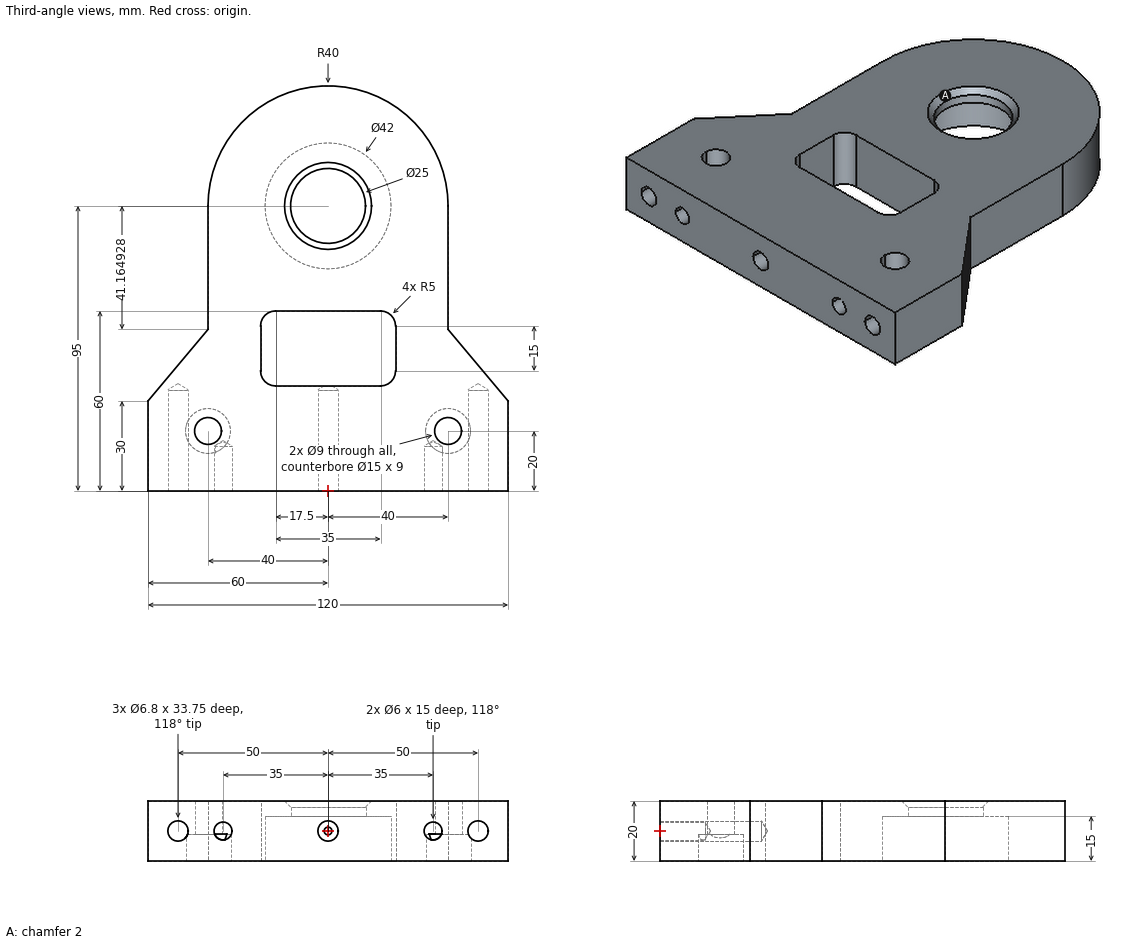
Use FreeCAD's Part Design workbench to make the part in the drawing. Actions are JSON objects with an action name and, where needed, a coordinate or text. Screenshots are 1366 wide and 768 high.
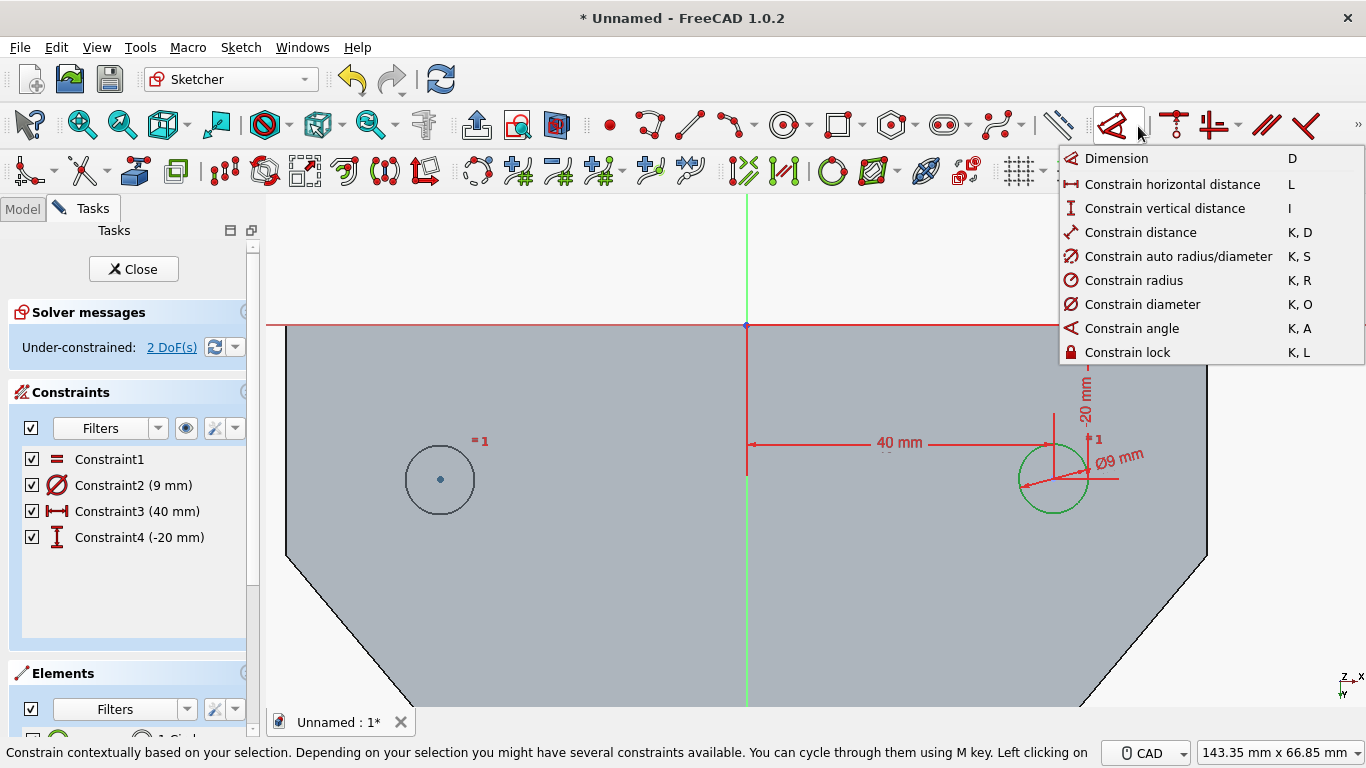
{"action": "left_click", "coordinate": [1212, 184]}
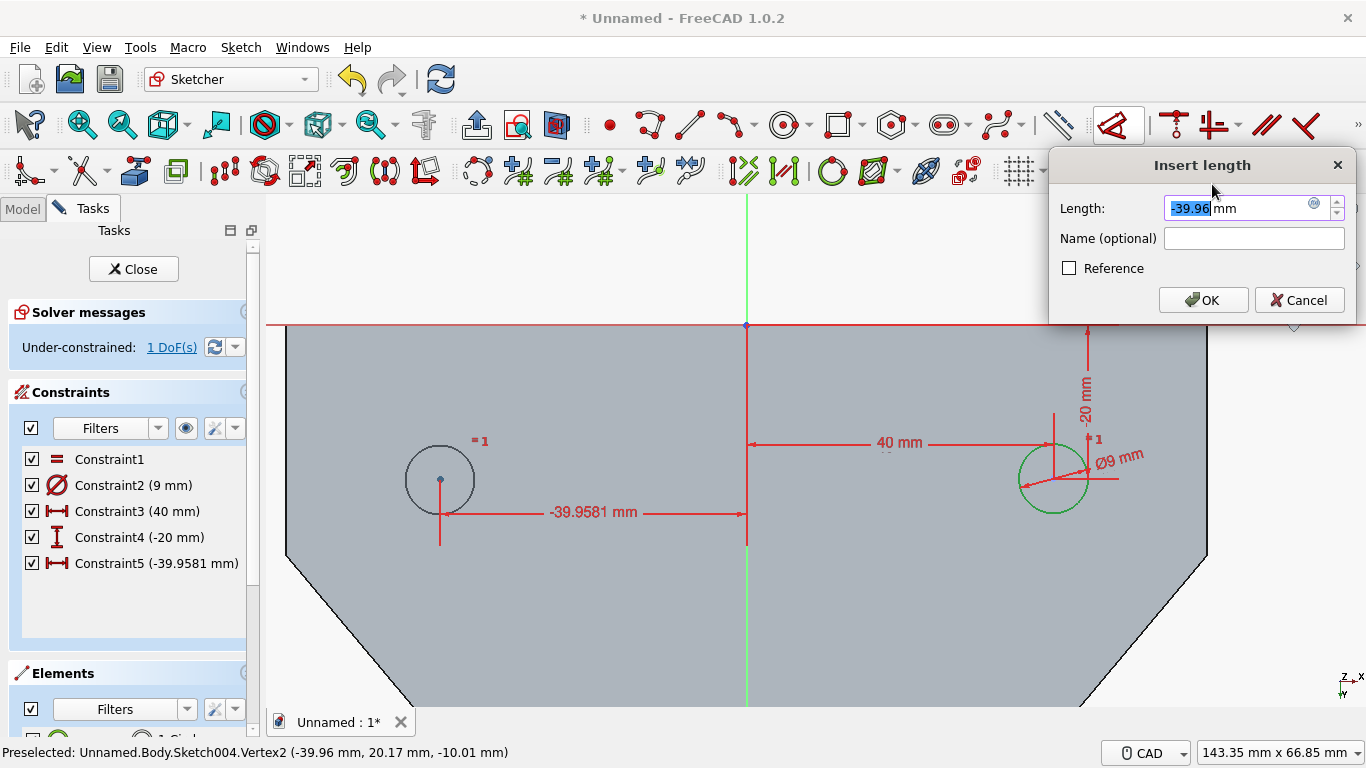
{"action": "type", "text": "-40"}
{"action": "key", "text": "Return"}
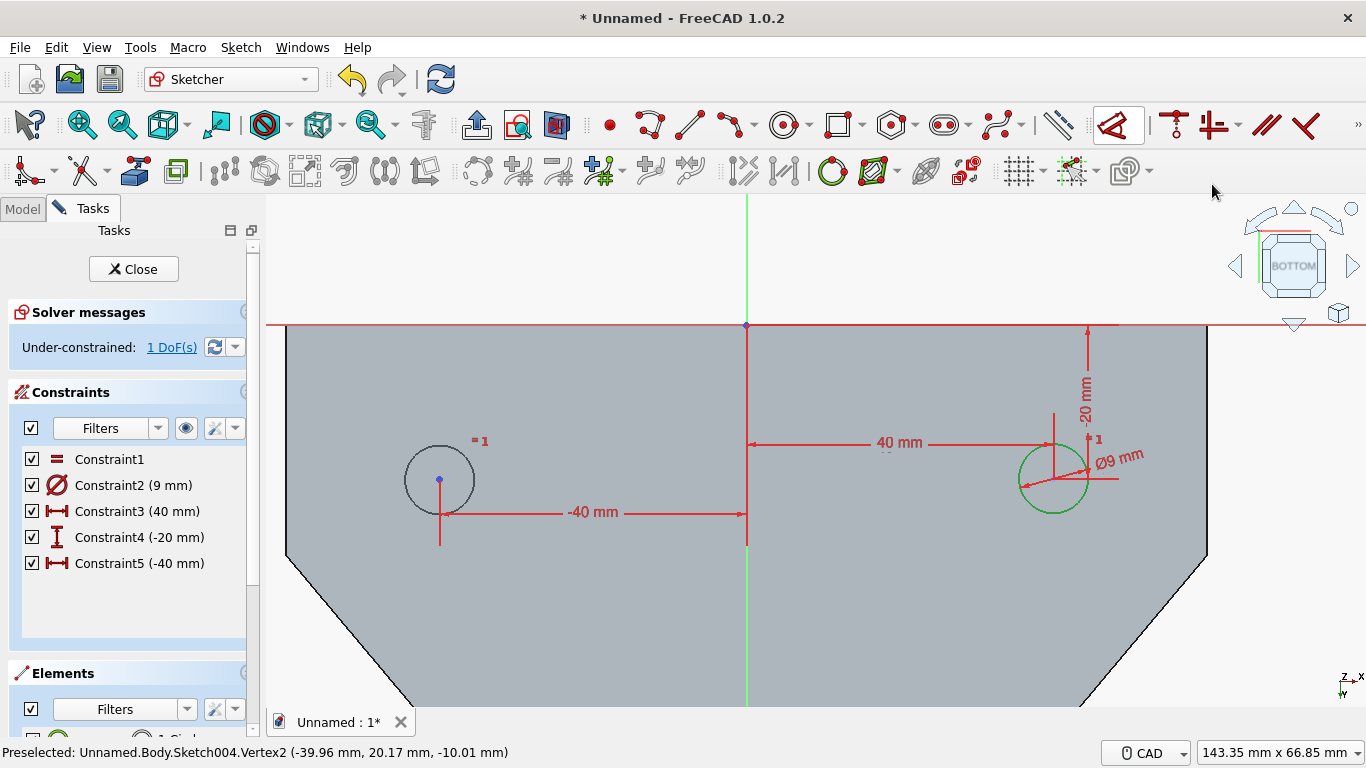
{"action": "left_click", "coordinate": [440, 480]}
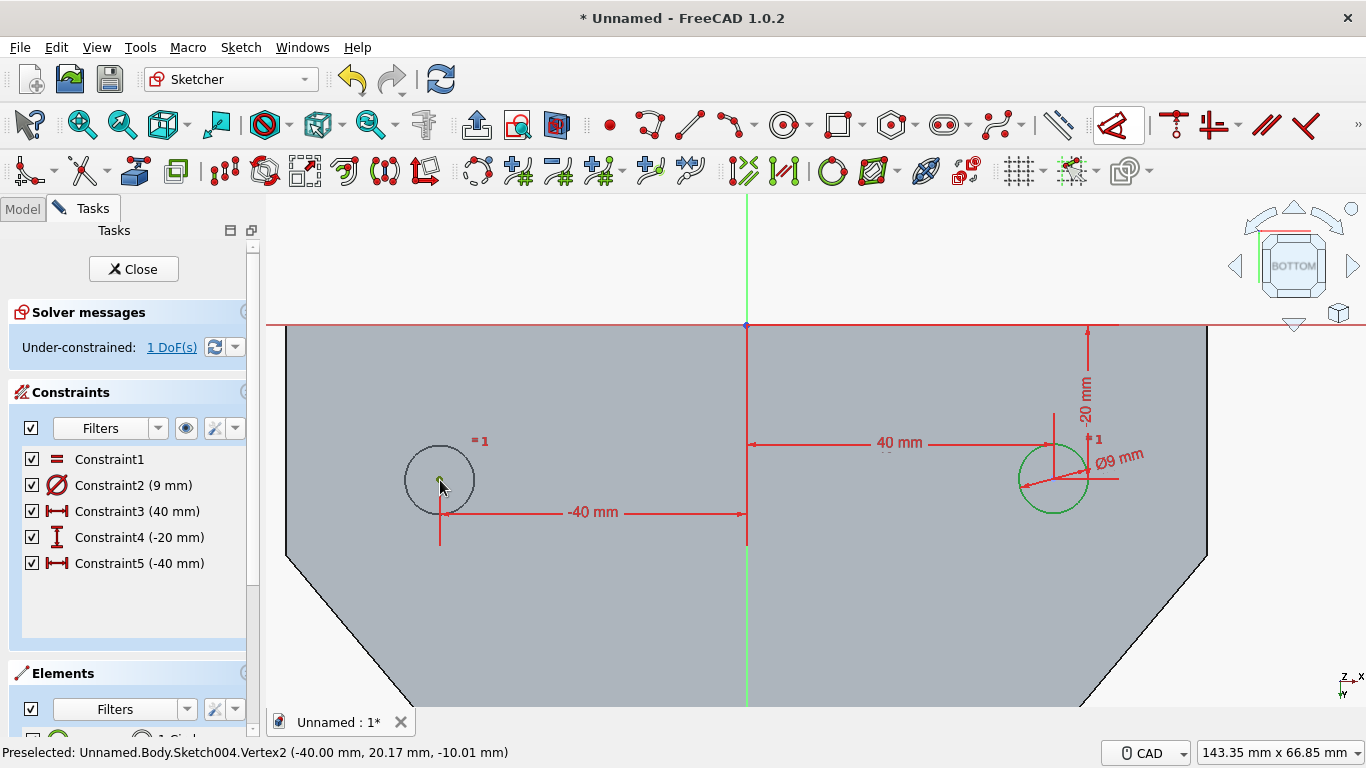
{"action": "key", "text": "i"}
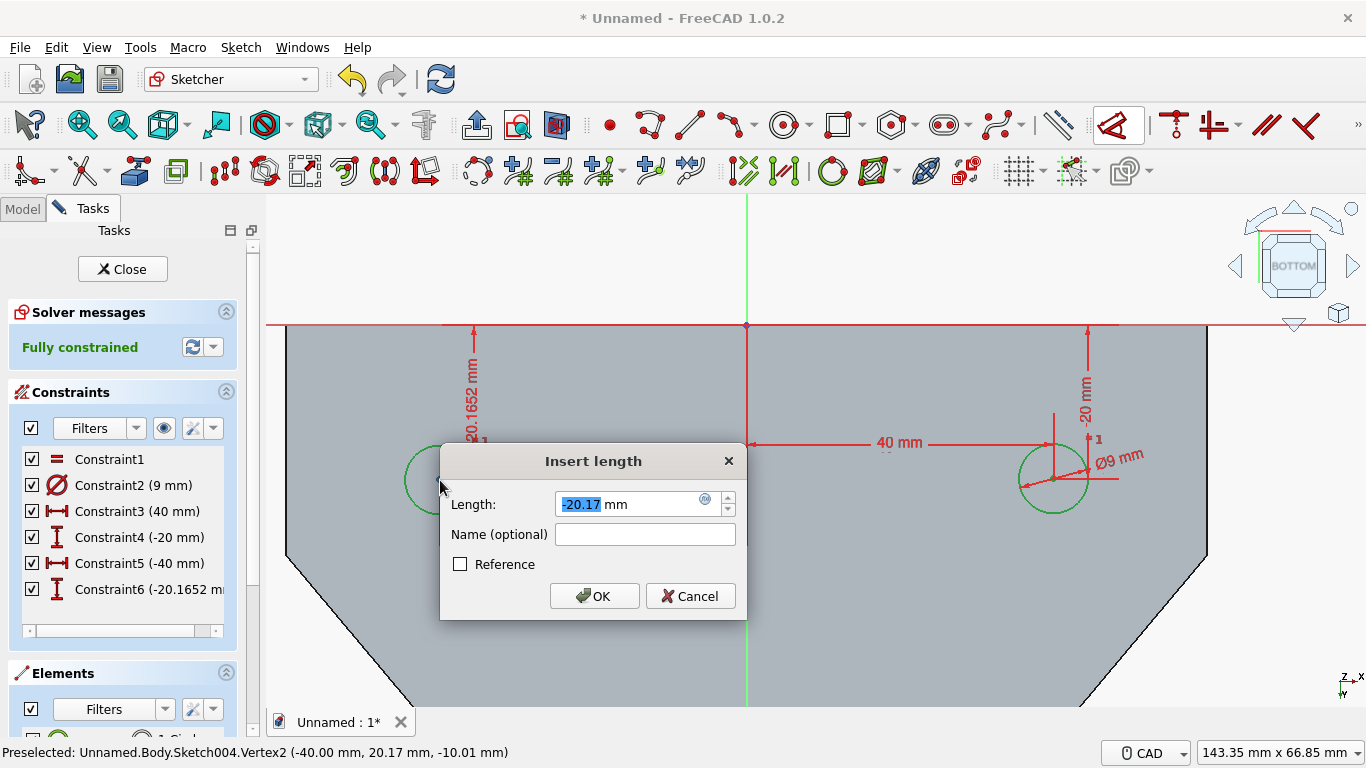
{"action": "type", "text": "-20"}
{"action": "key", "text": "Return"}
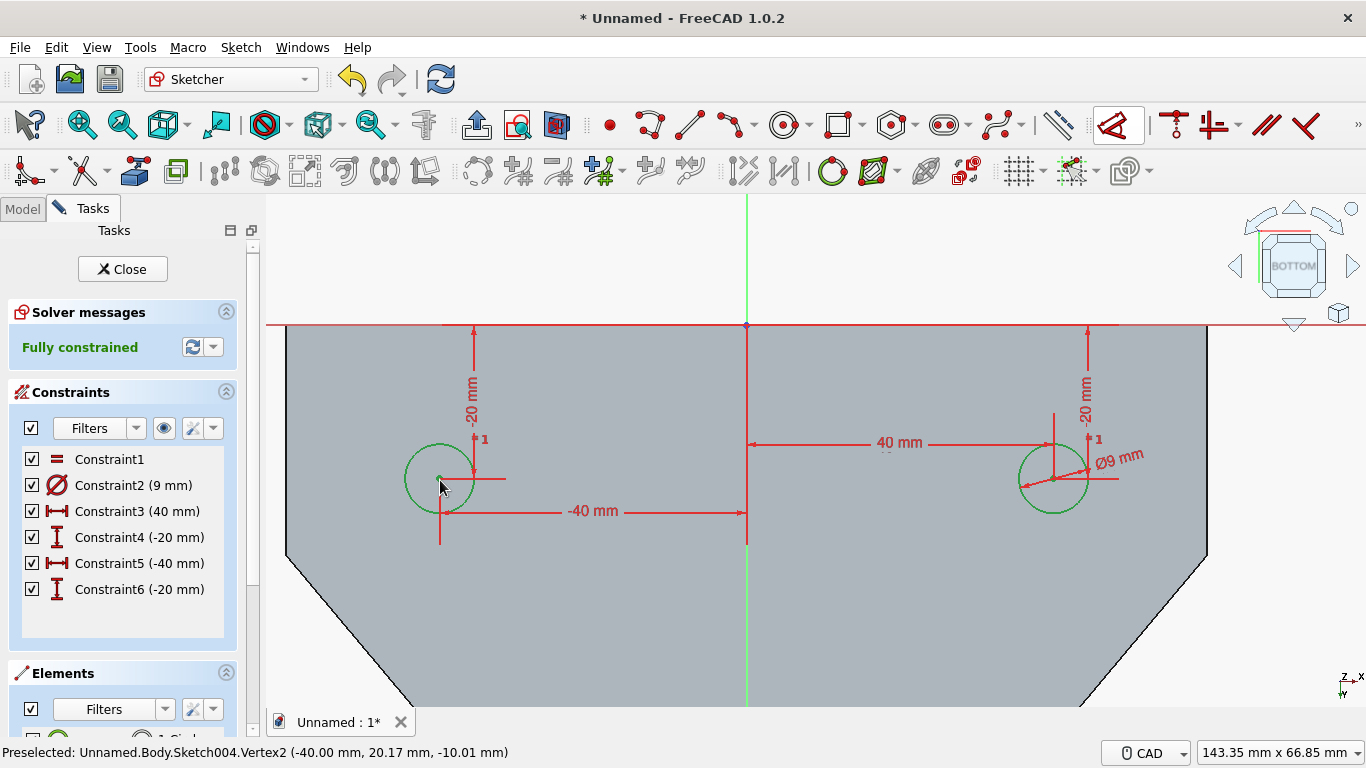
{"action": "left_click", "coordinate": [123, 269]}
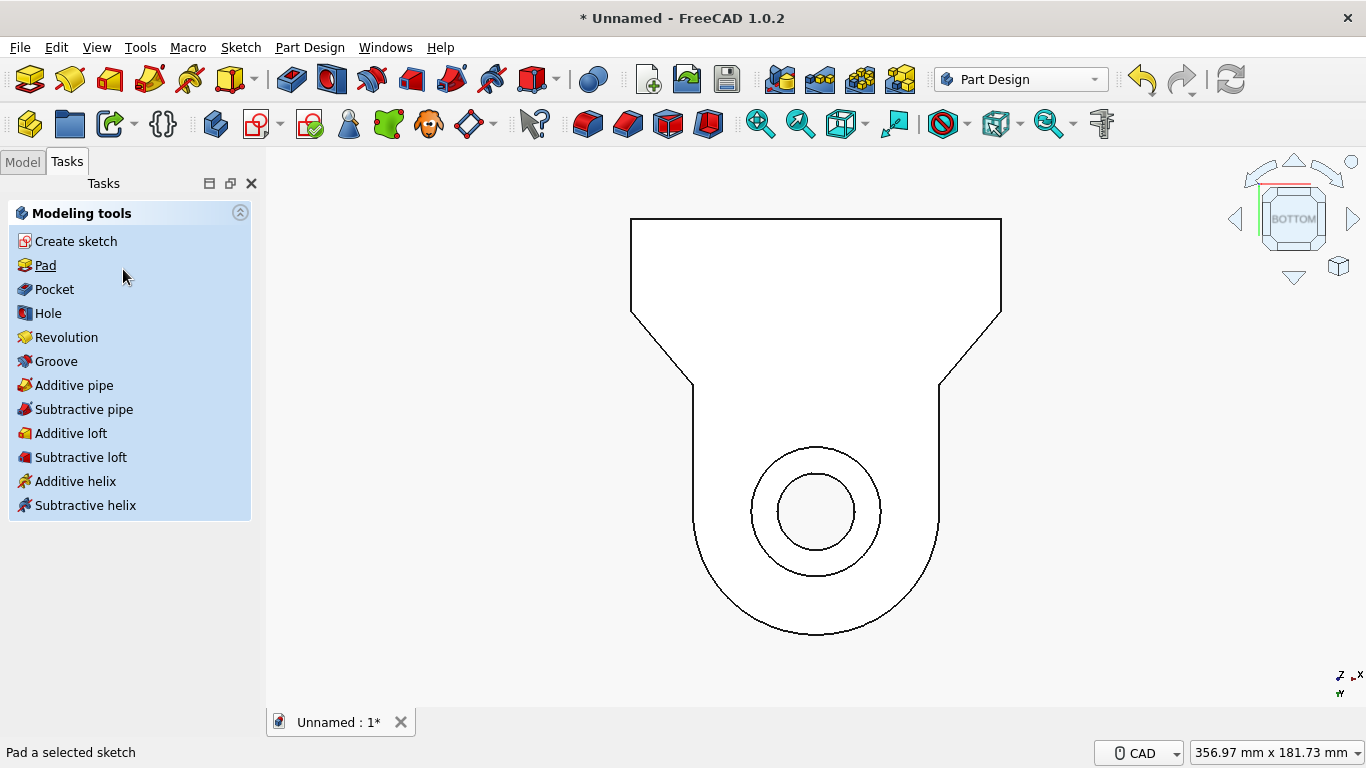
{"action": "left_click", "coordinate": [332, 80]}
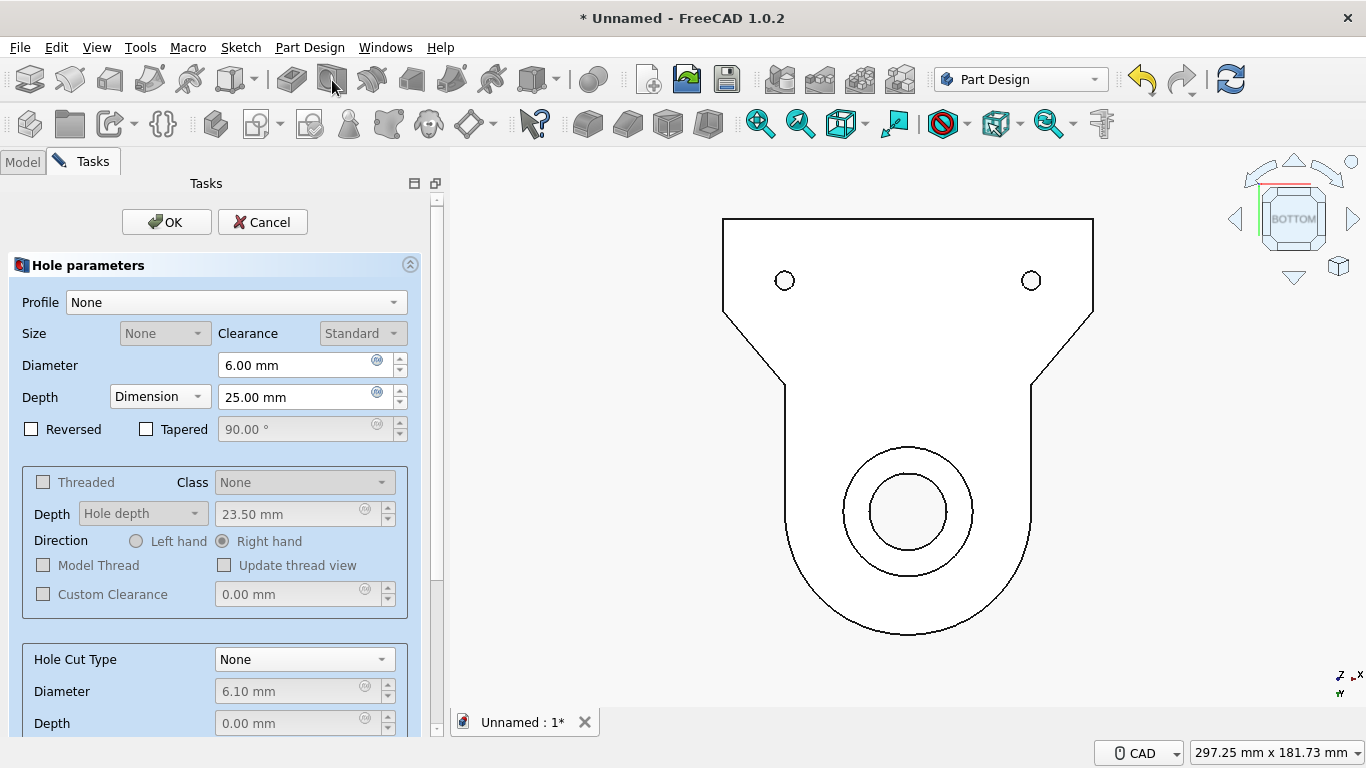
{"action": "triple_click", "coordinate": [305, 365]}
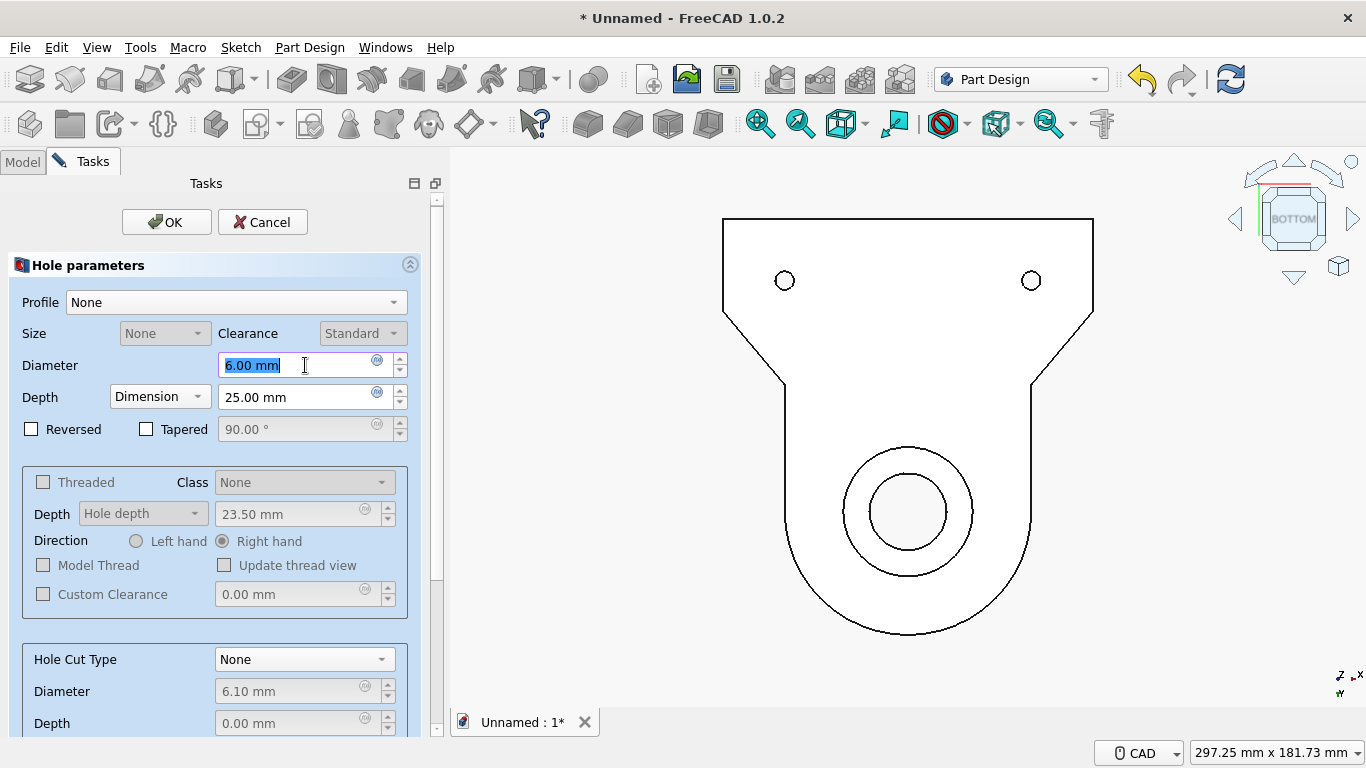
{"action": "type", "text": "9"}
{"action": "key", "text": "Tab"}